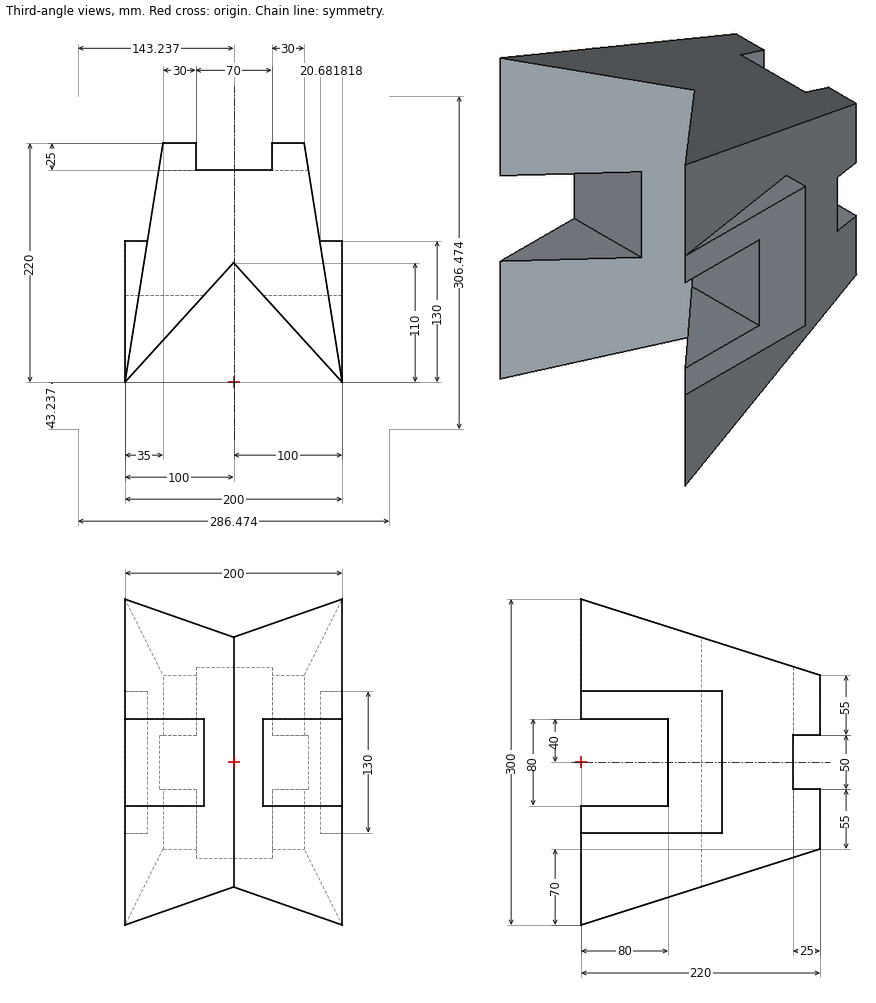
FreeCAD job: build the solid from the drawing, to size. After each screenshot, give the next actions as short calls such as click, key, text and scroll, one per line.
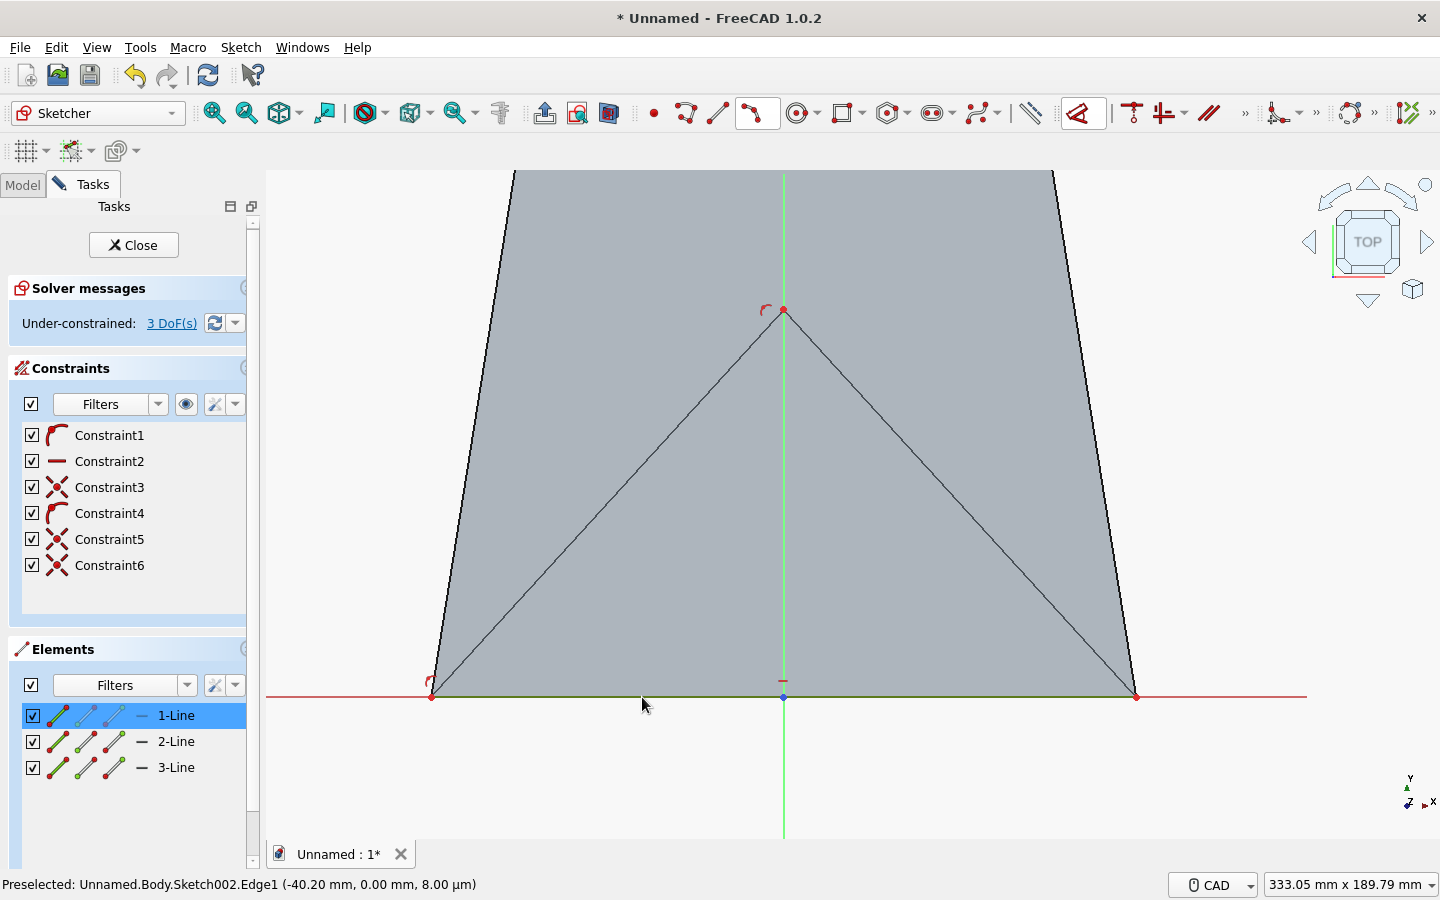
key(l)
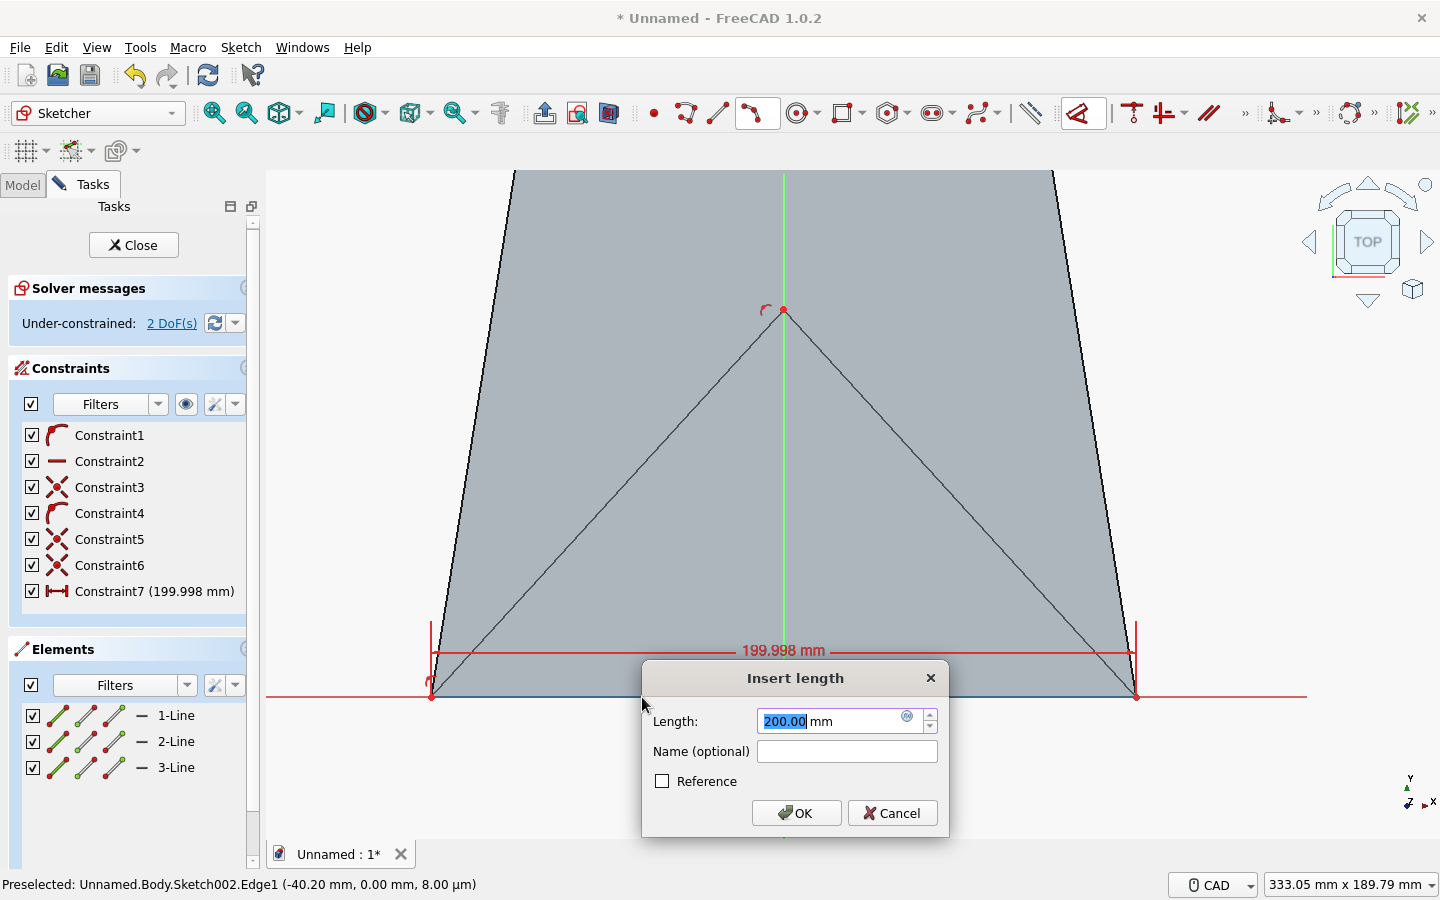
text(200)
key(Return)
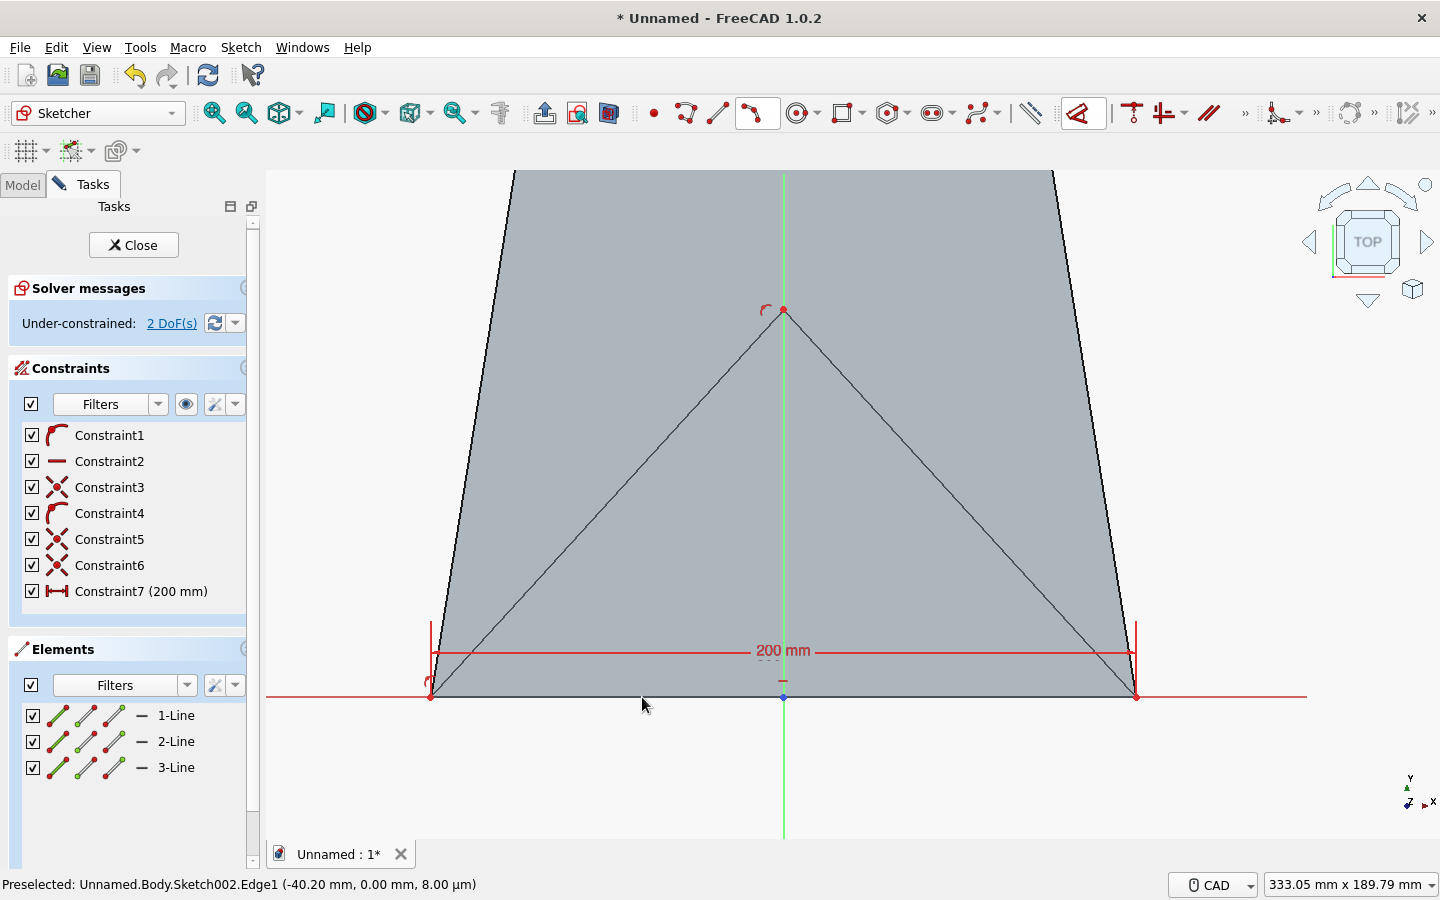
click(431, 697)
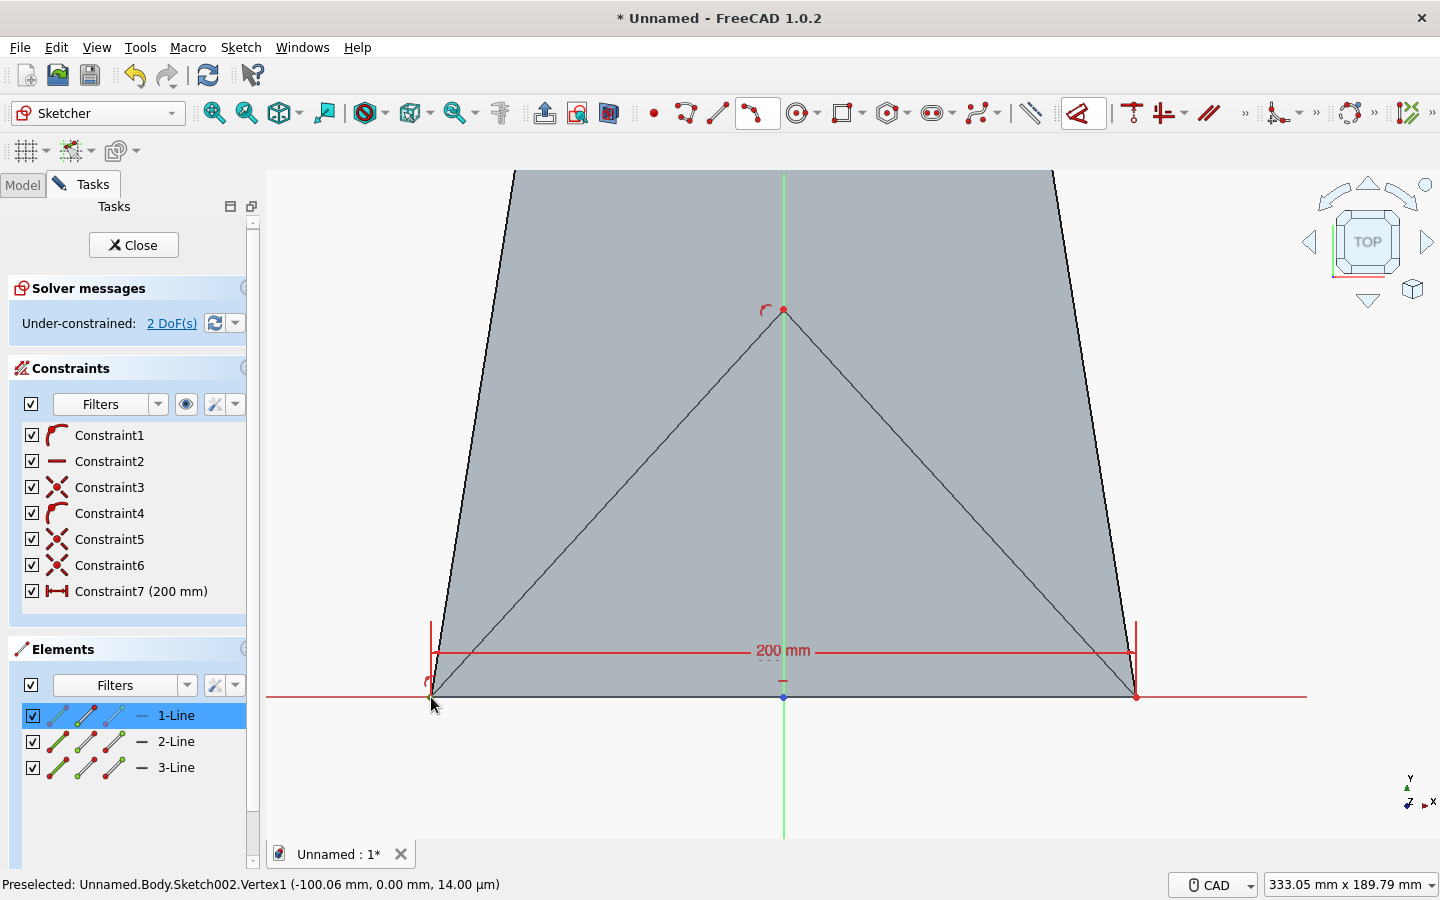
key(l)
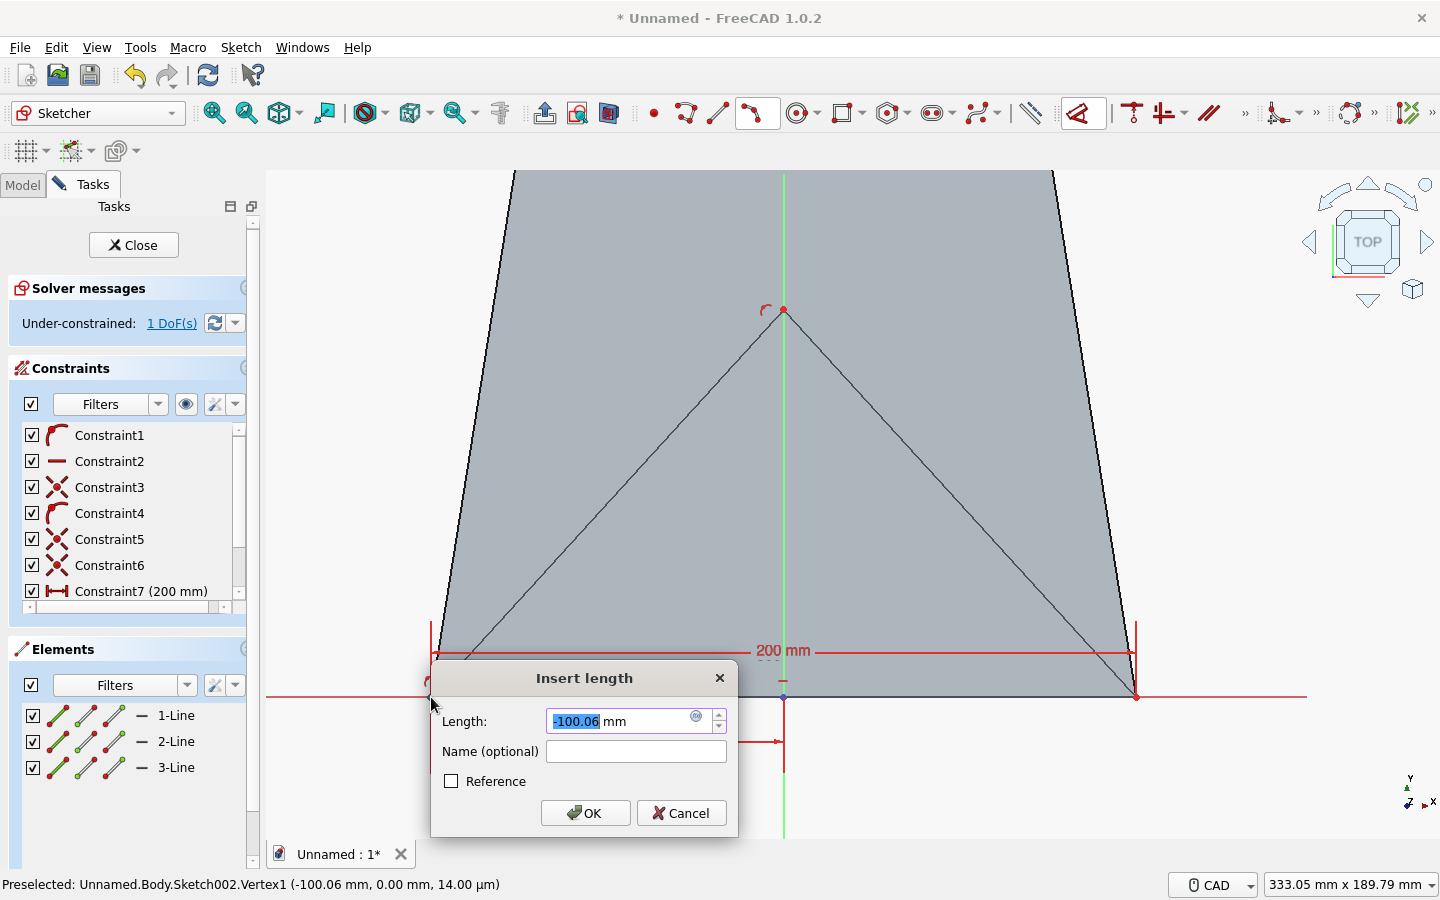
text(-100)
key(Return)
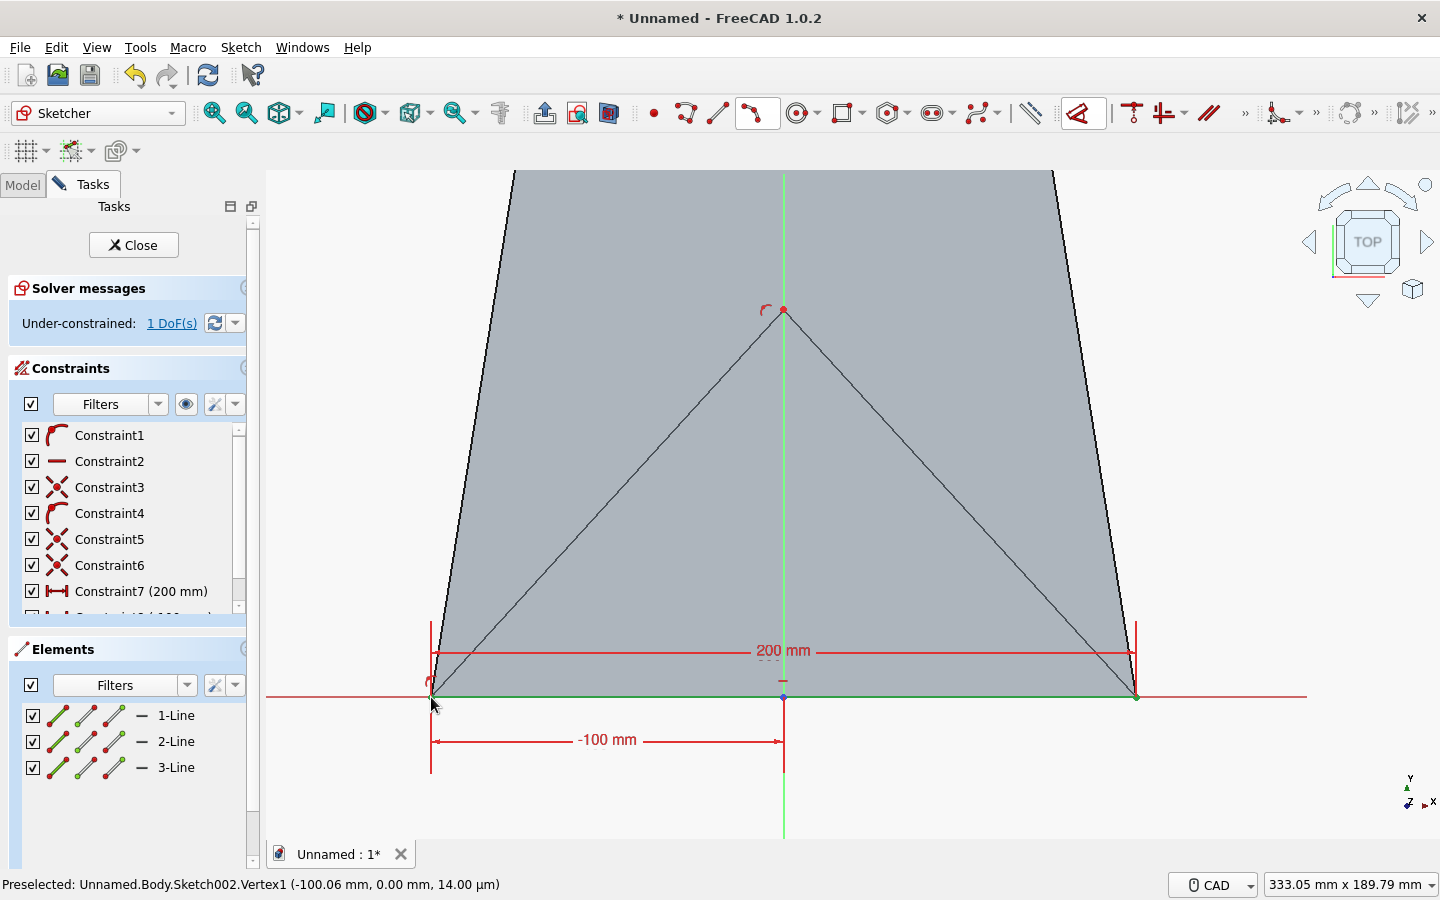
click(784, 310)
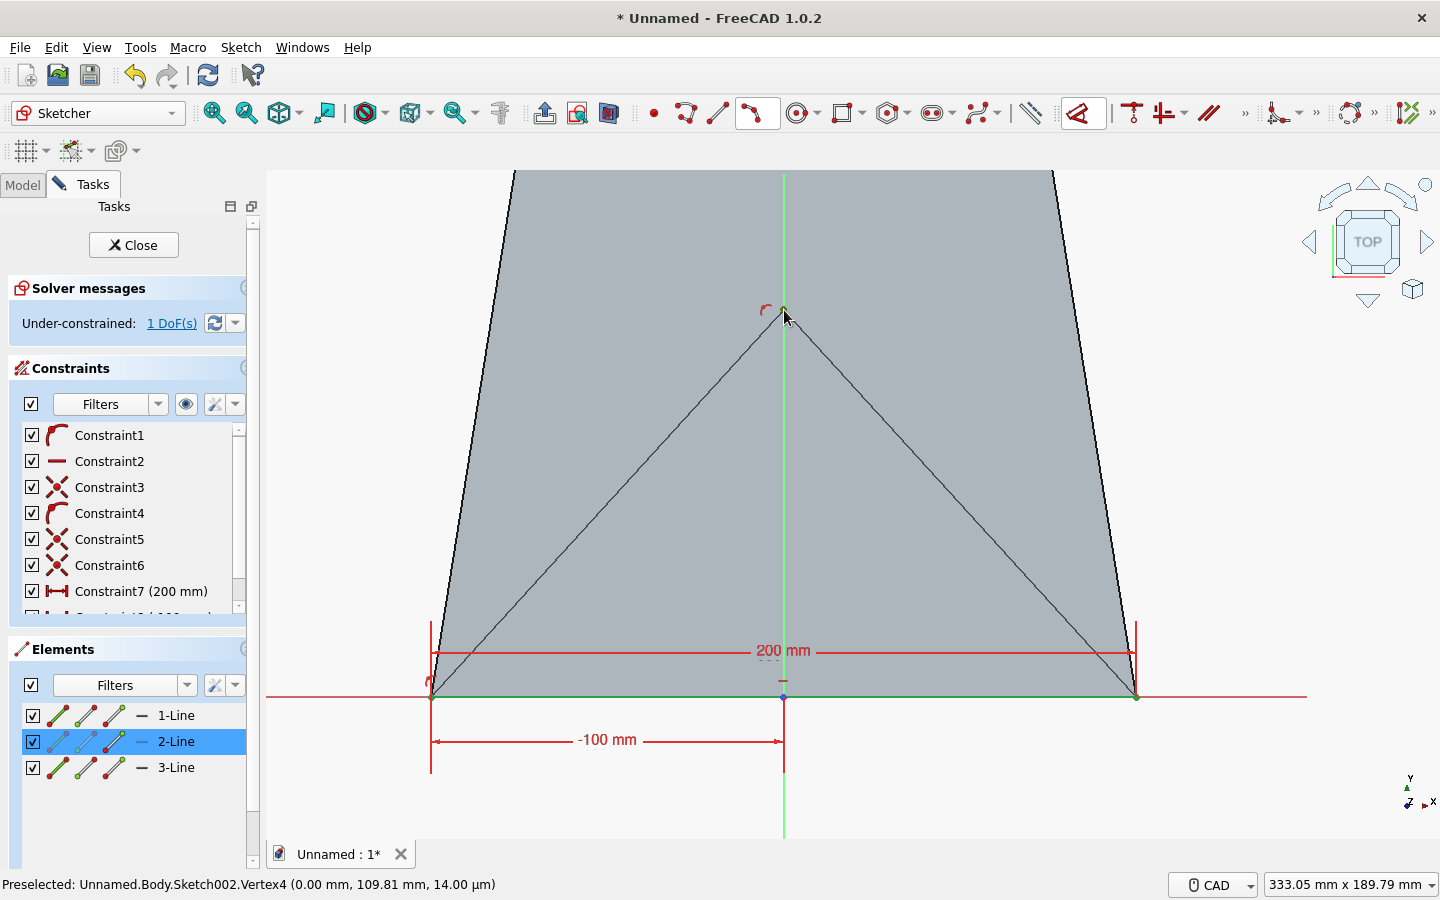
click(1100, 114)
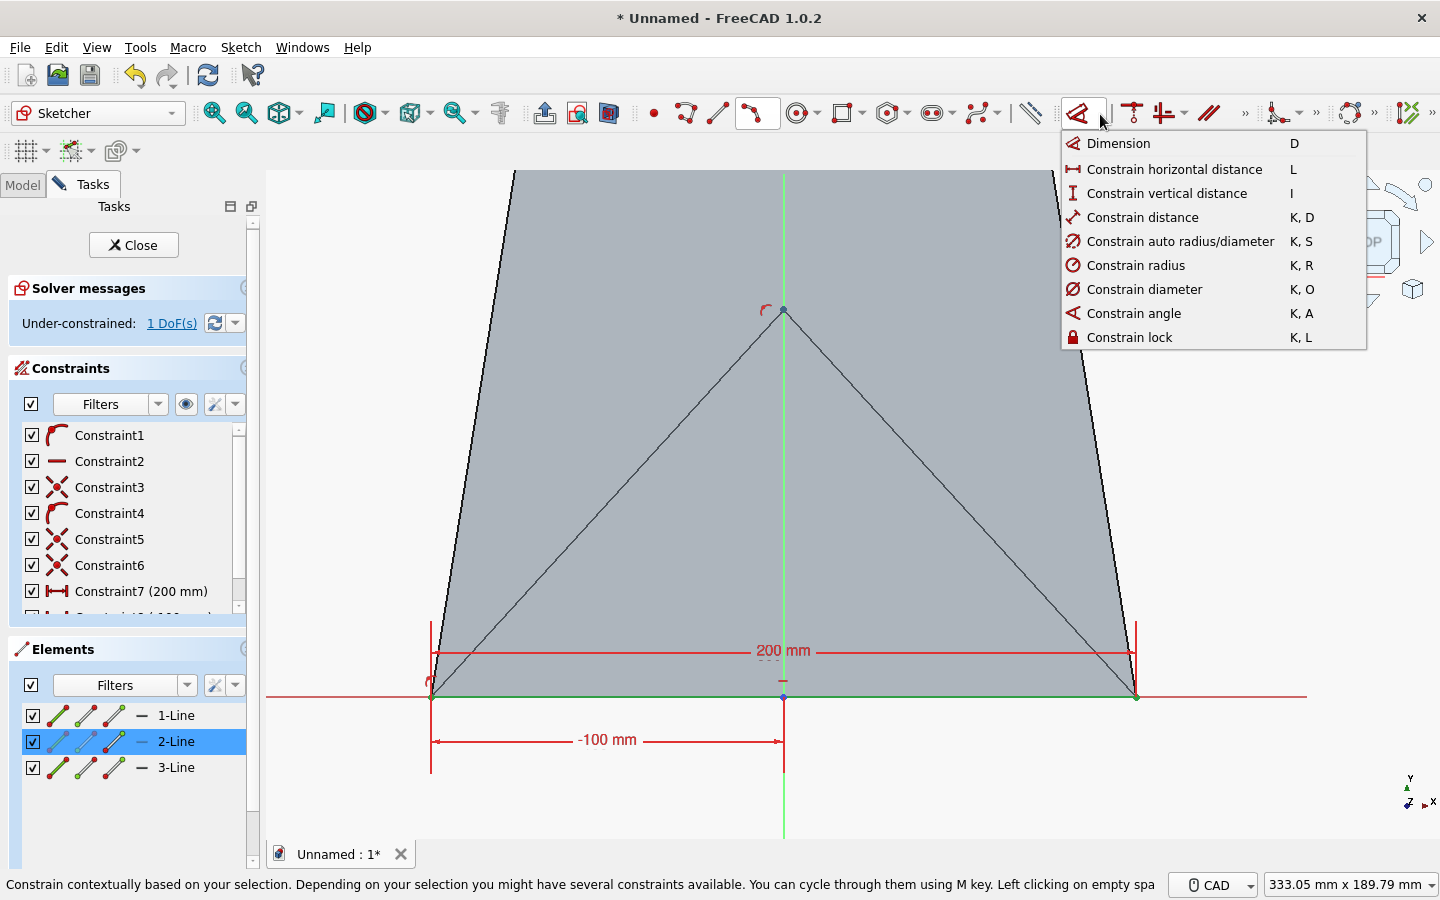
click(1214, 193)